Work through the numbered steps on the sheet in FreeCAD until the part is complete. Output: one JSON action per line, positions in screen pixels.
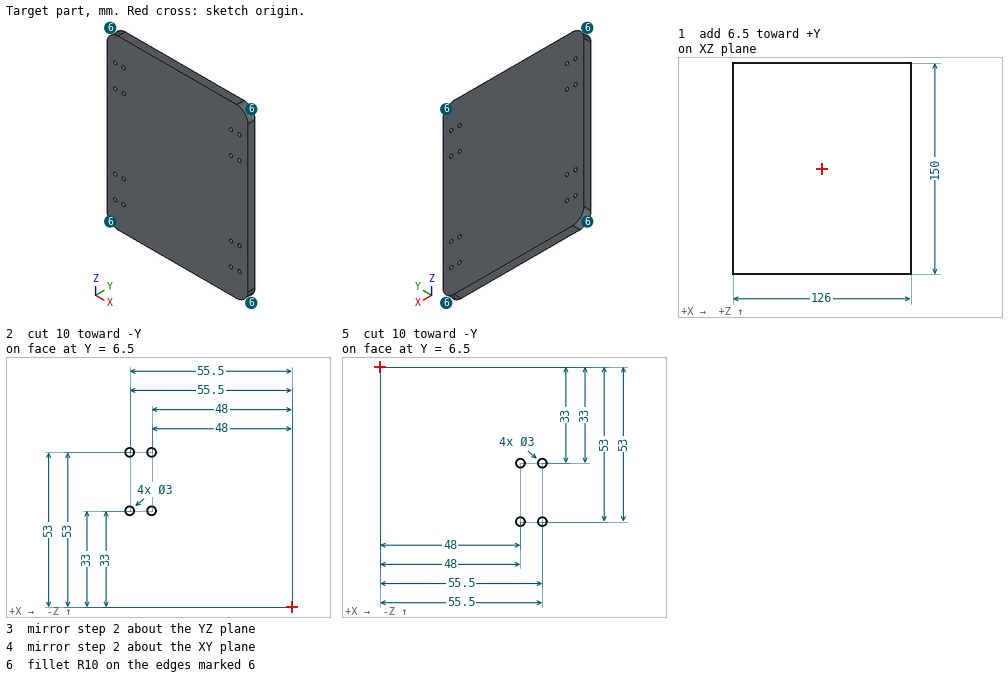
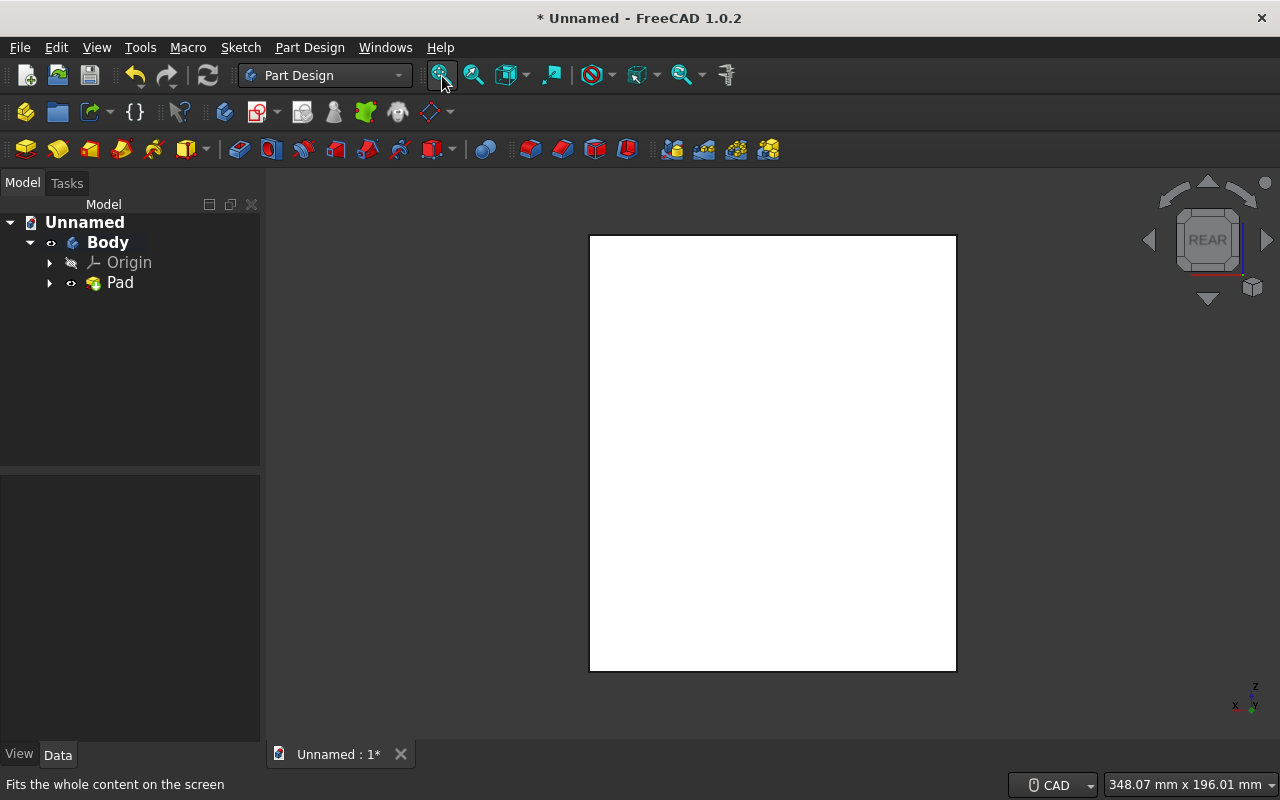
{"action": "left_click", "coordinate": [773, 452]}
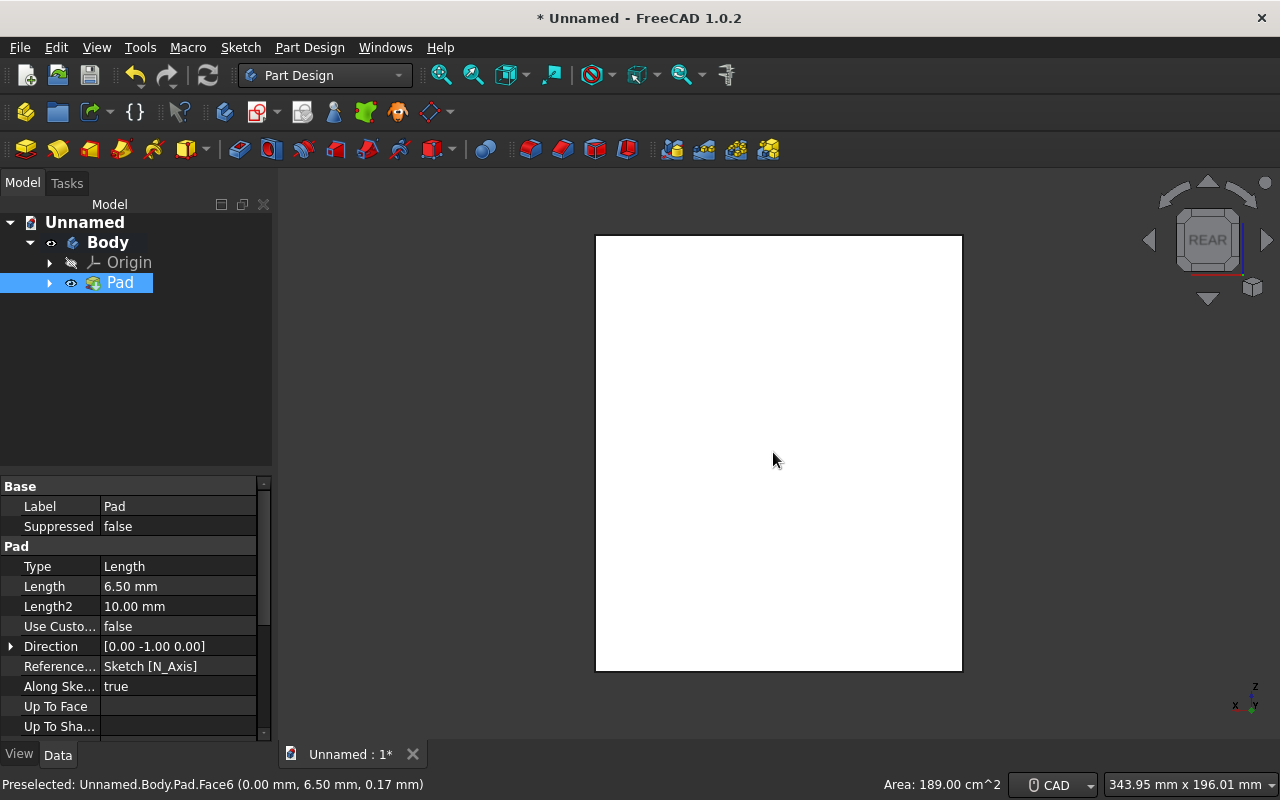
{"action": "left_click", "coordinate": [258, 112]}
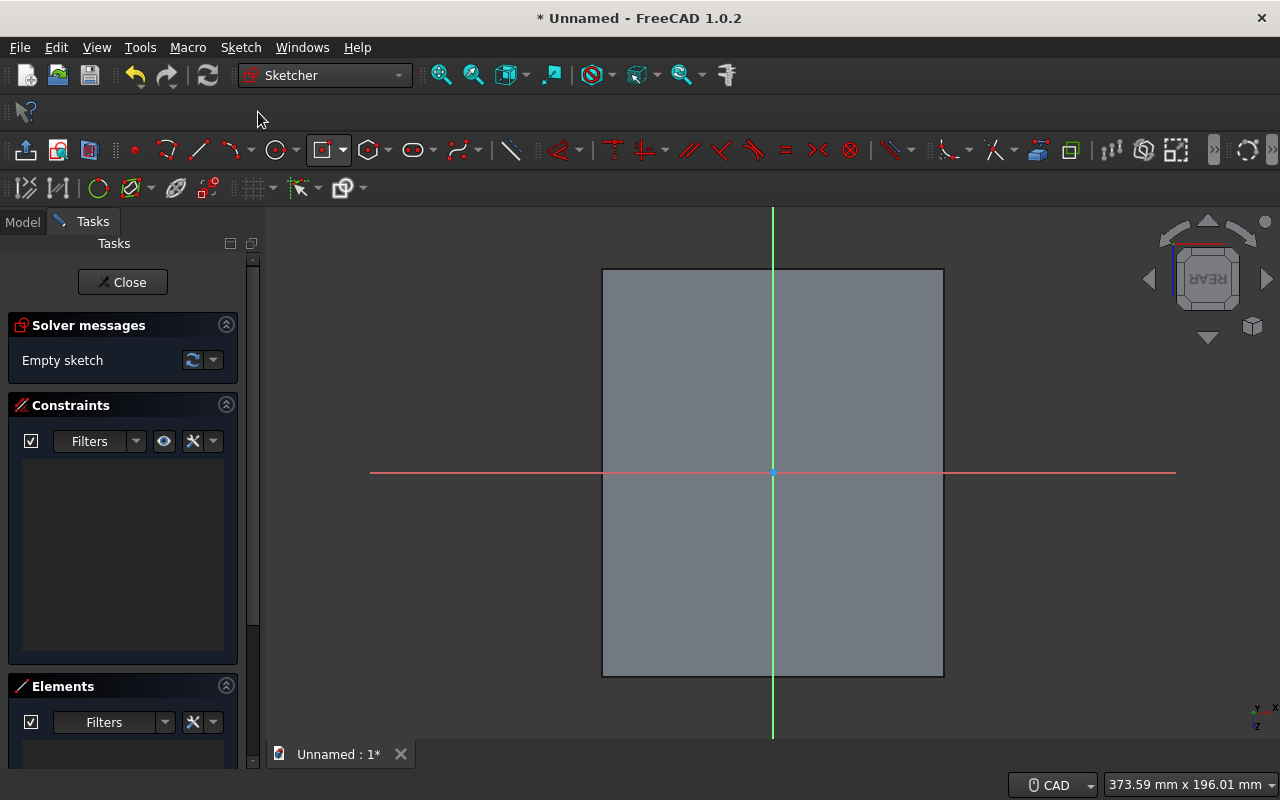
{"action": "scroll", "coordinate": [688, 339], "scroll_direction": "up", "scroll_amount": 4}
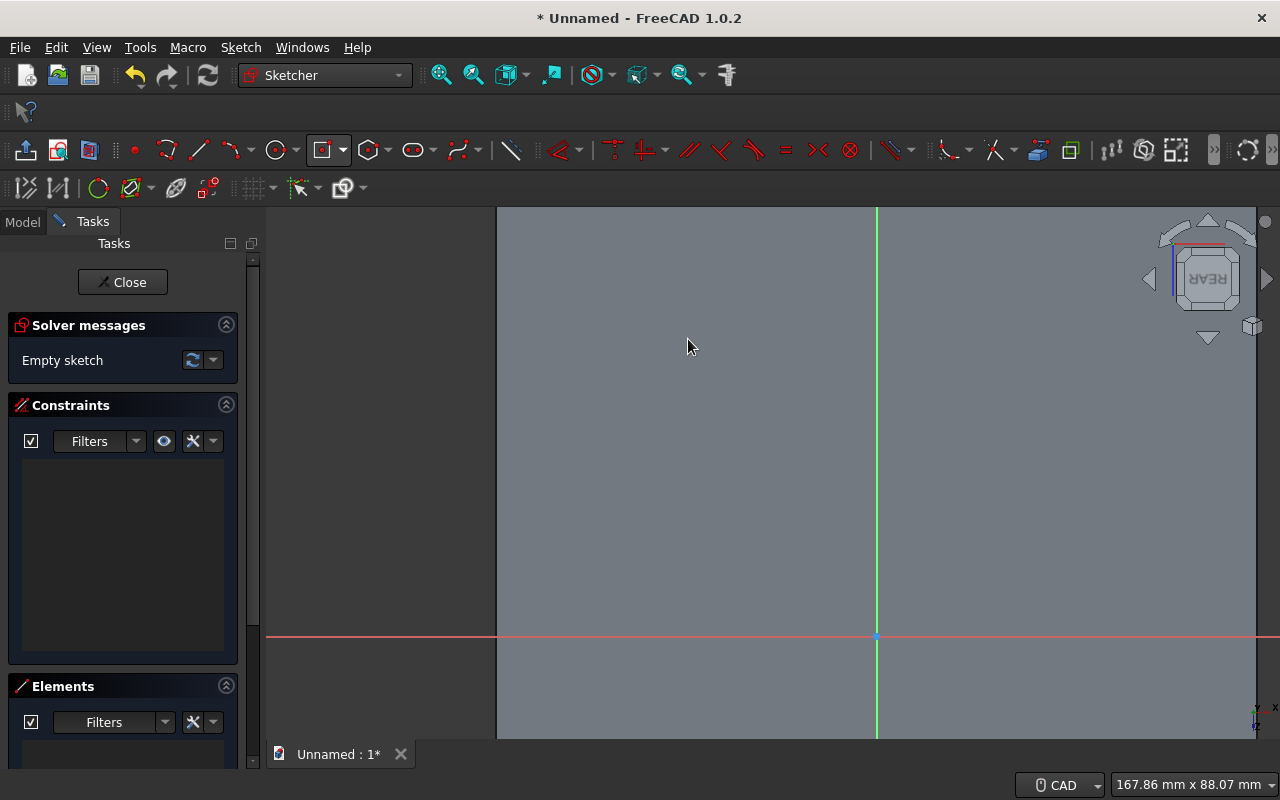
{"action": "left_click", "coordinate": [276, 150]}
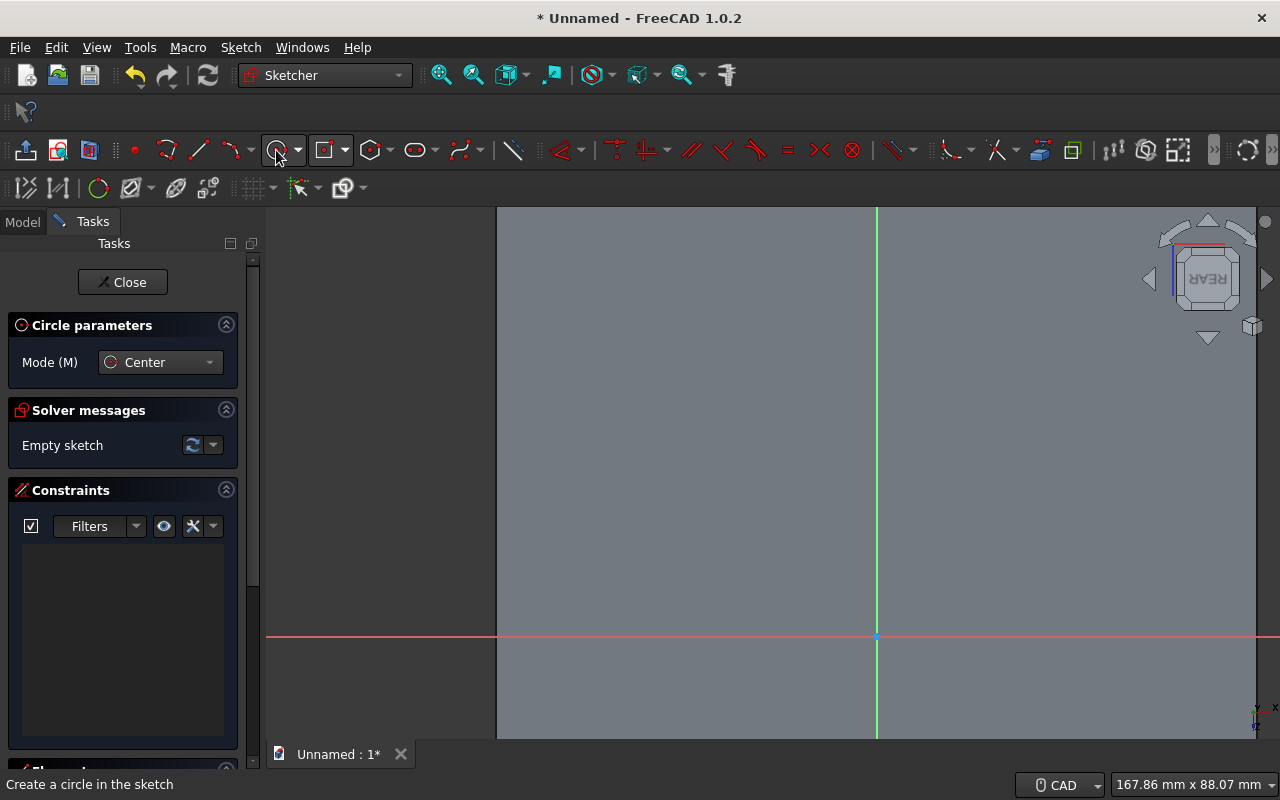
{"action": "scroll", "coordinate": [541, 438], "scroll_direction": "up", "scroll_amount": 5}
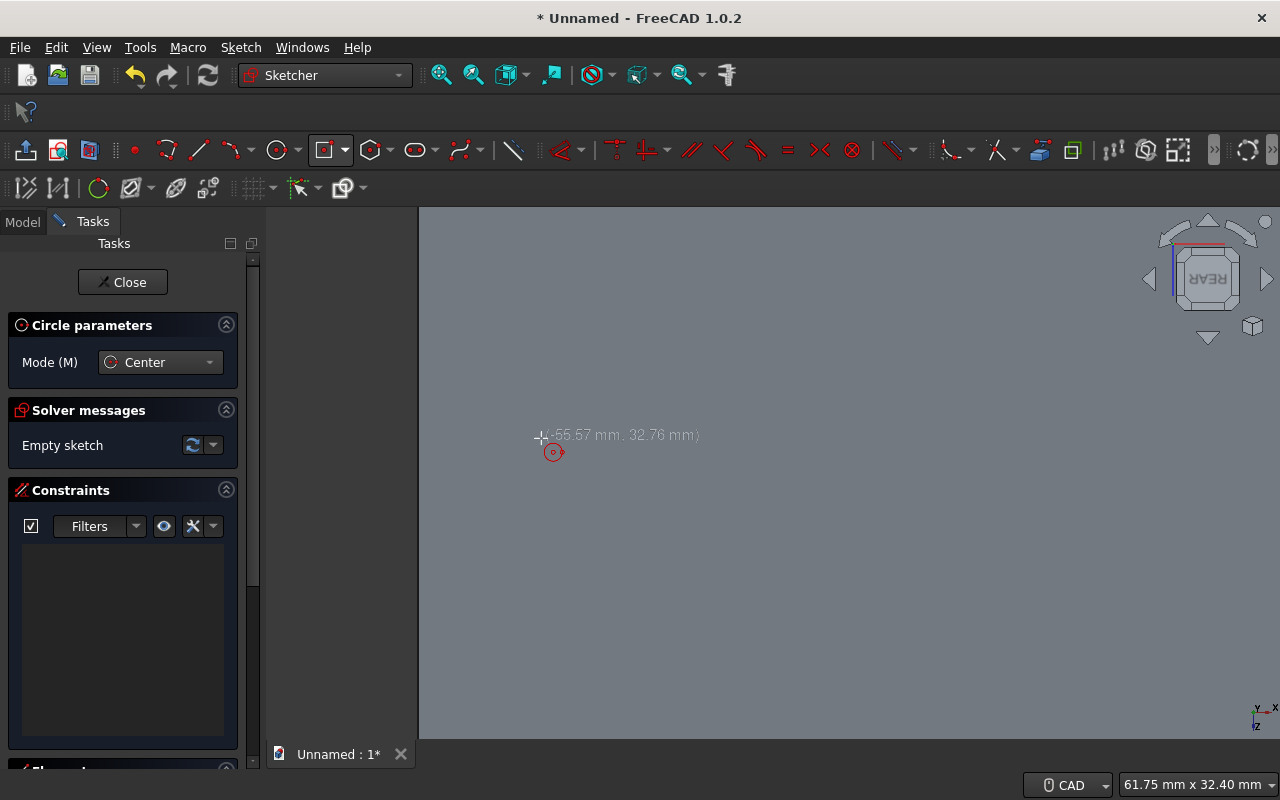
{"action": "left_click", "coordinate": [542, 436]}
{"action": "left_click", "coordinate": [559, 419]}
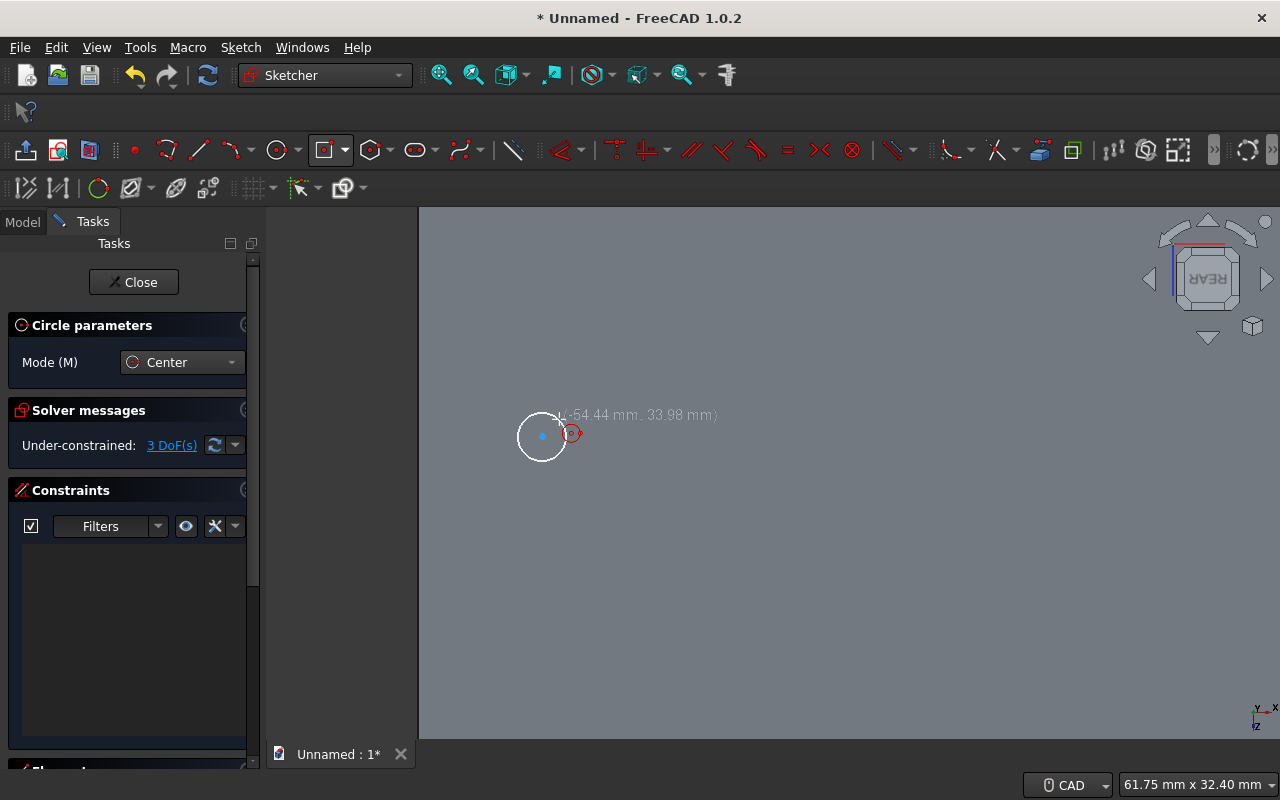
{"action": "left_click", "coordinate": [665, 436]}
{"action": "left_click", "coordinate": [682, 419]}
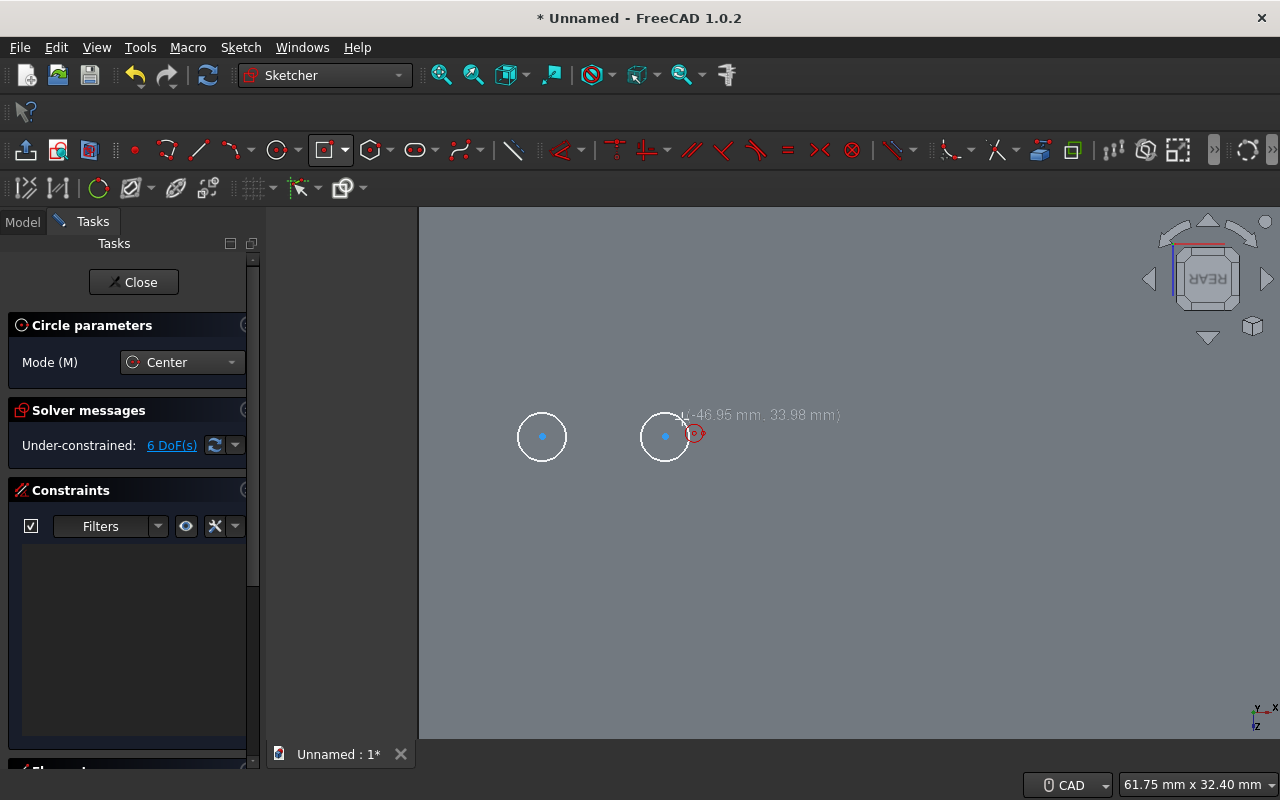
{"action": "scroll", "coordinate": [541, 440], "scroll_direction": "down", "scroll_amount": 5}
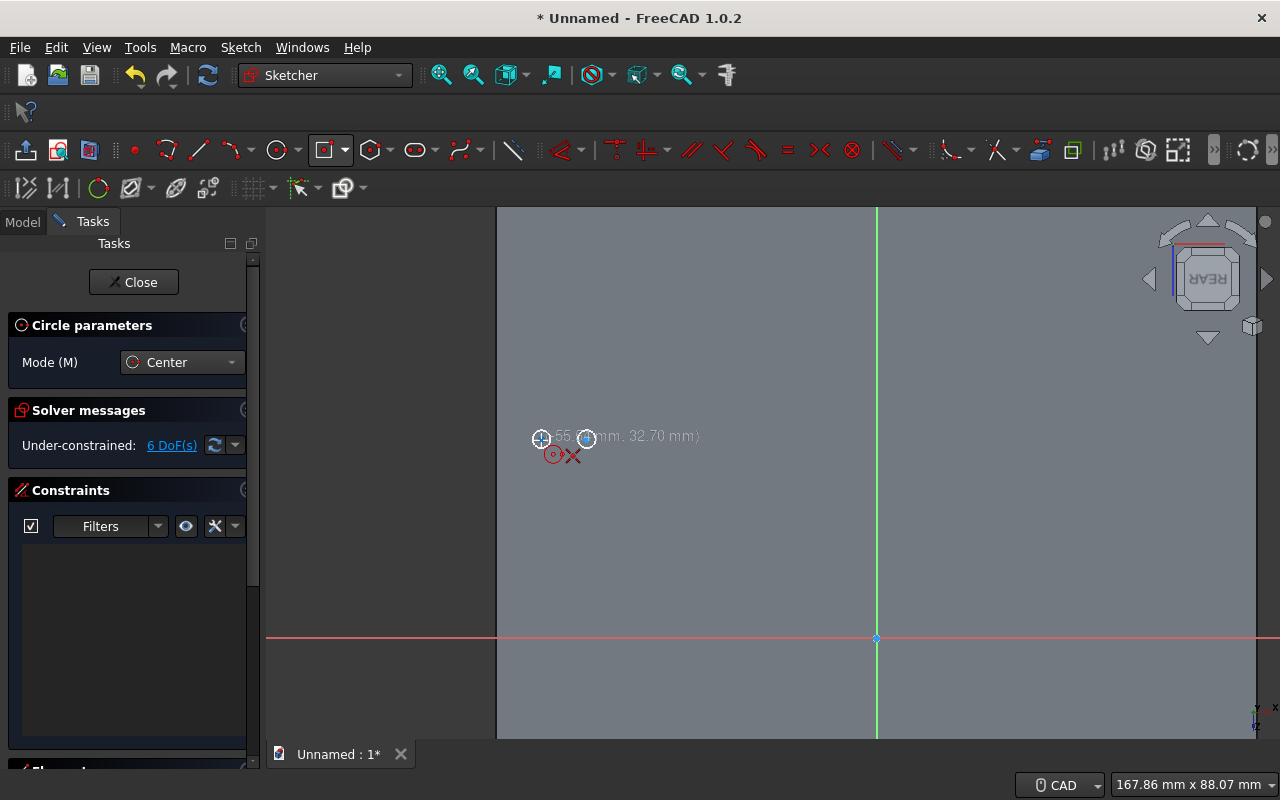
{"action": "scroll", "coordinate": [587, 318], "scroll_direction": "up", "scroll_amount": 5}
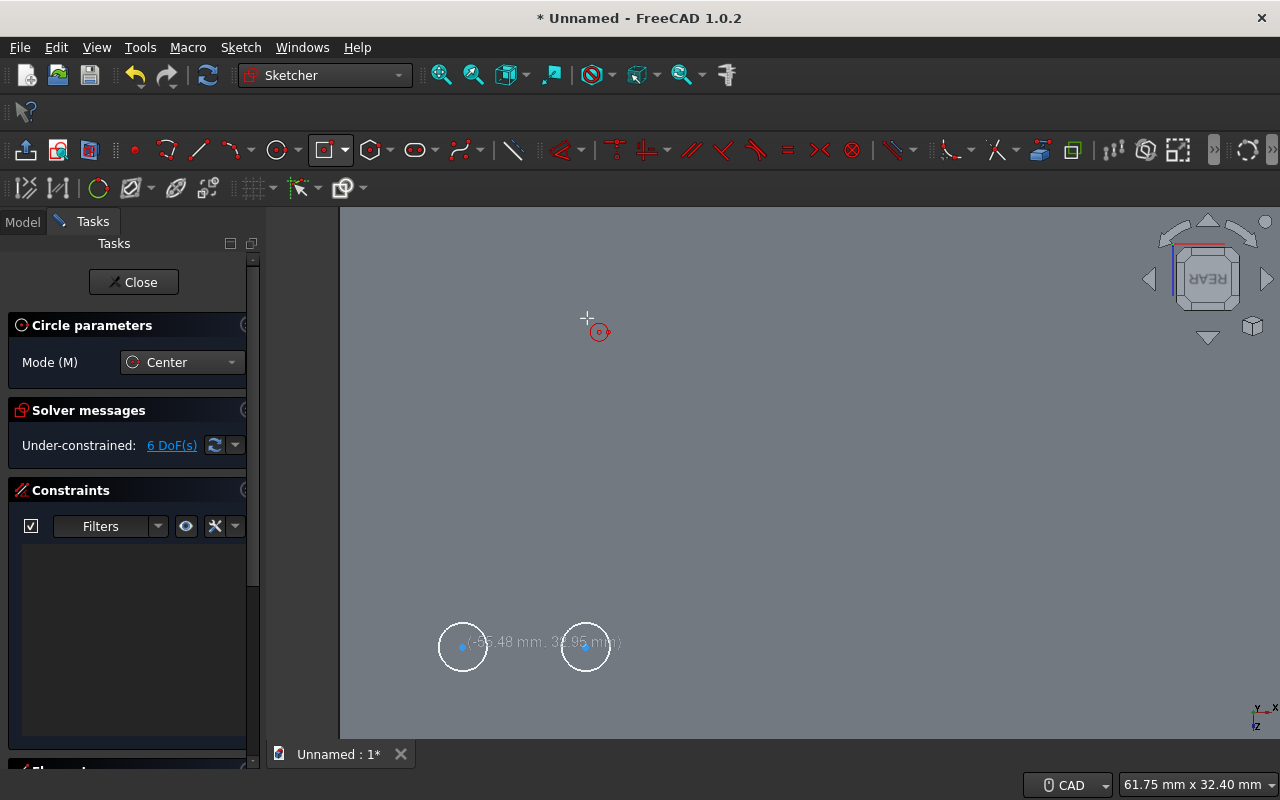
{"action": "left_click", "coordinate": [586, 318]}
{"action": "left_click", "coordinate": [603, 300]}